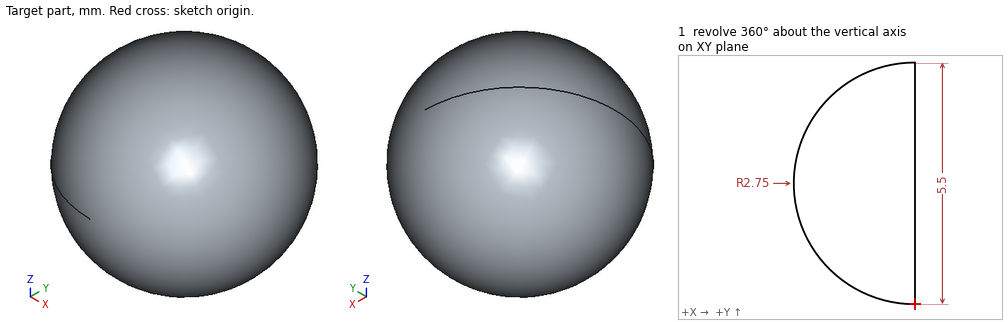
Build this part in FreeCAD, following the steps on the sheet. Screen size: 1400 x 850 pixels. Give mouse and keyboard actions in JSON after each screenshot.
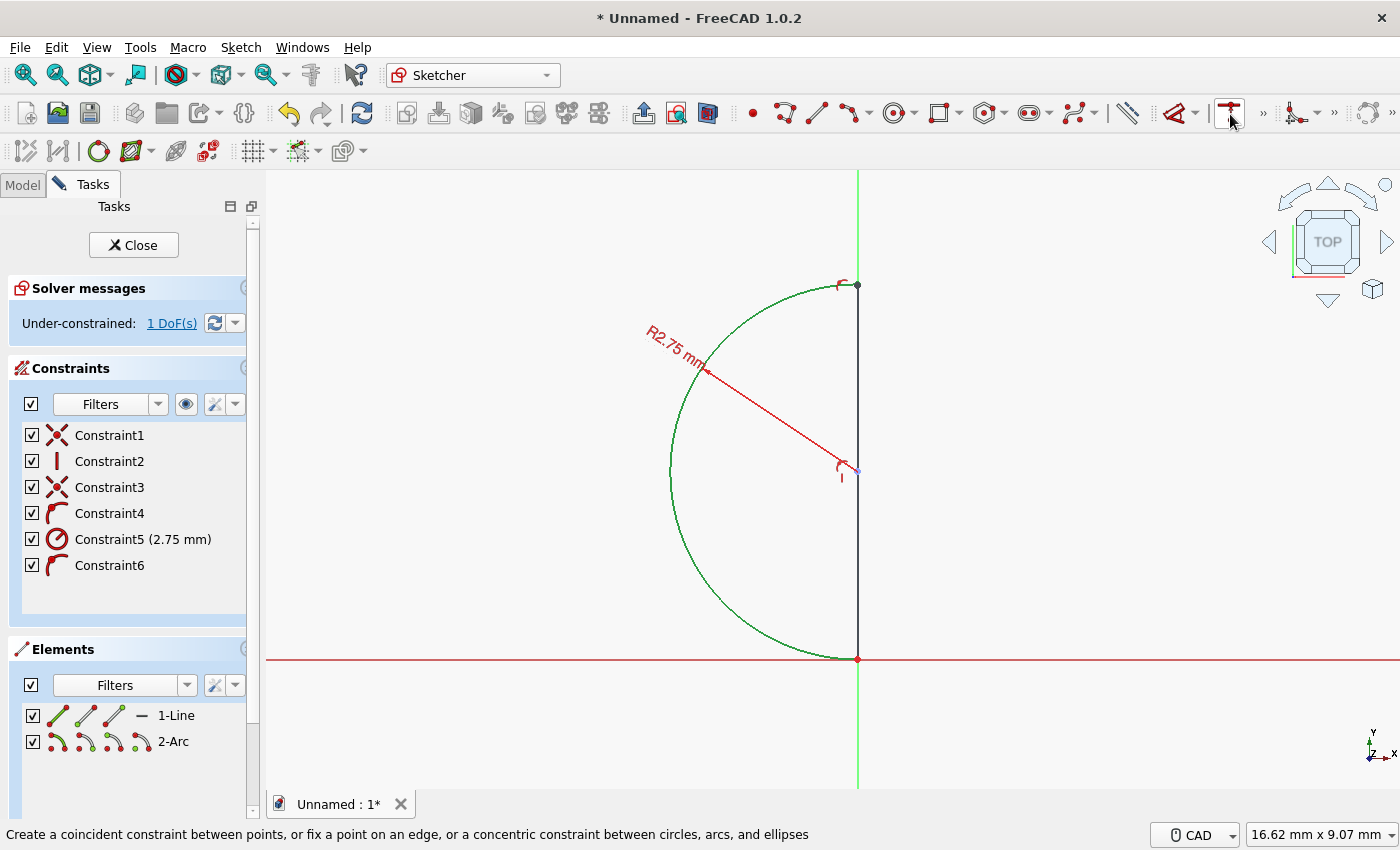
{"action": "left_click", "coordinate": [1174, 114]}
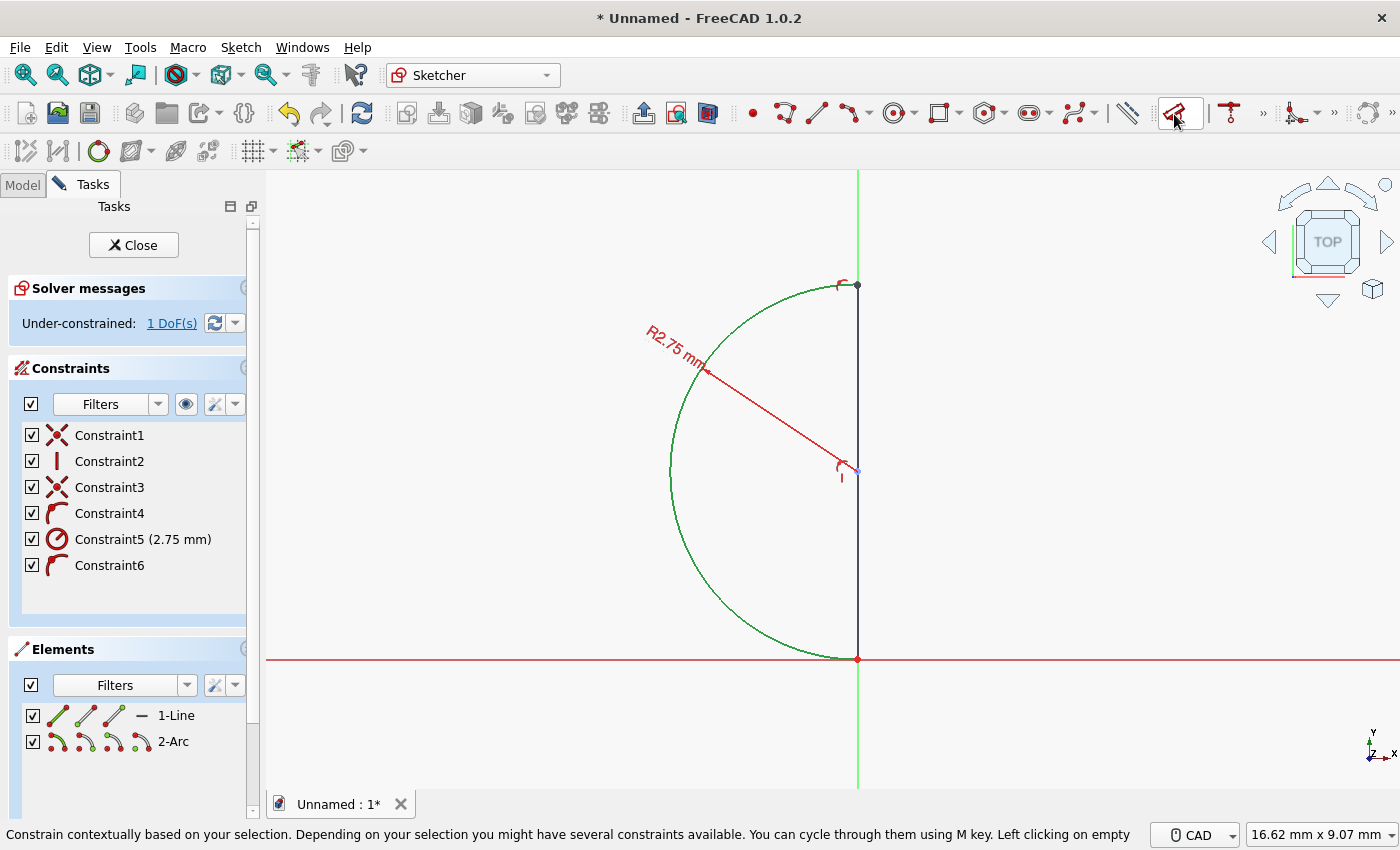
{"action": "left_click", "coordinate": [858, 547]}
{"action": "left_click", "coordinate": [892, 473]}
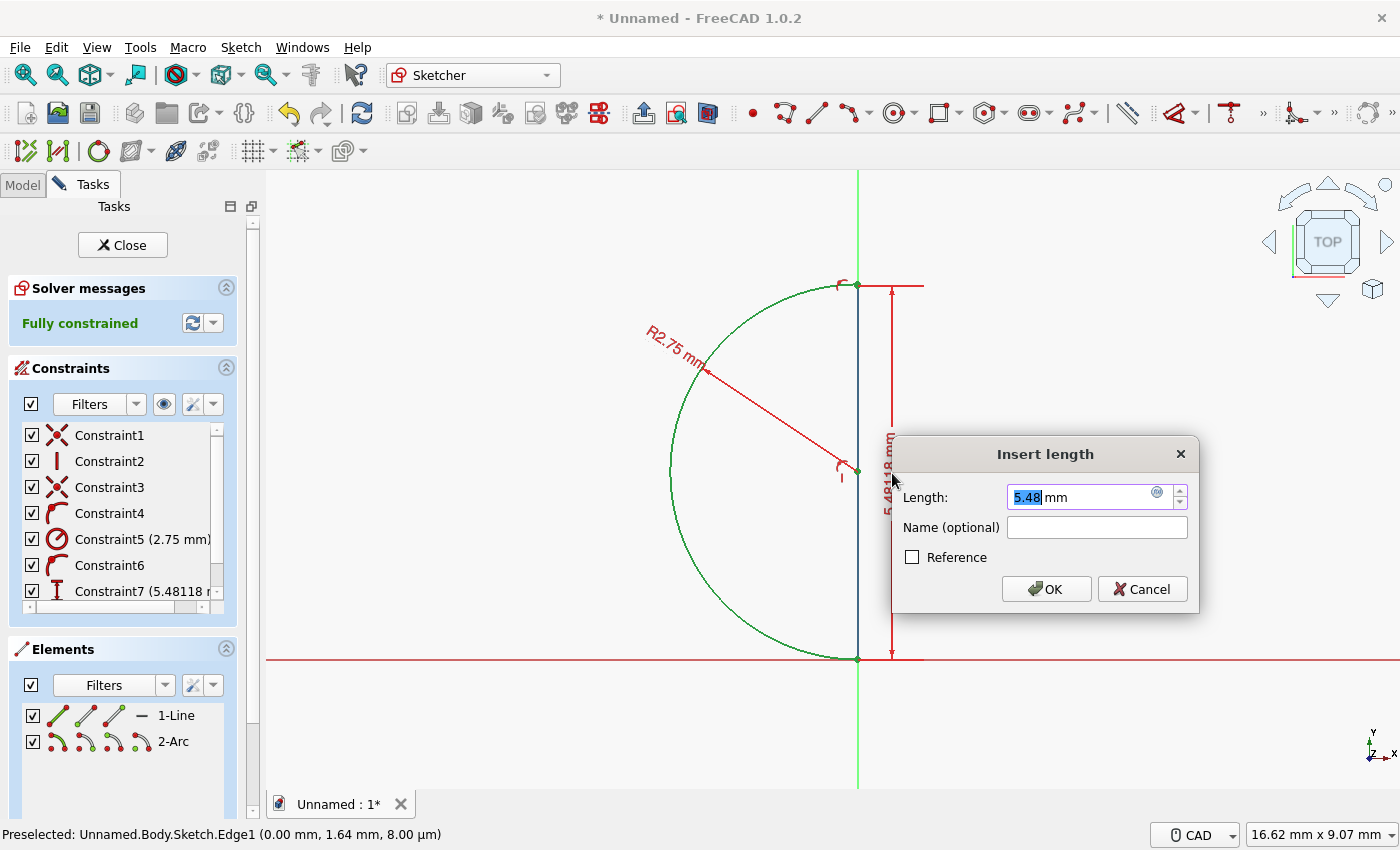
{"action": "type", "text": "5.5"}
{"action": "key", "text": "Return"}
{"action": "key", "text": "Escape"}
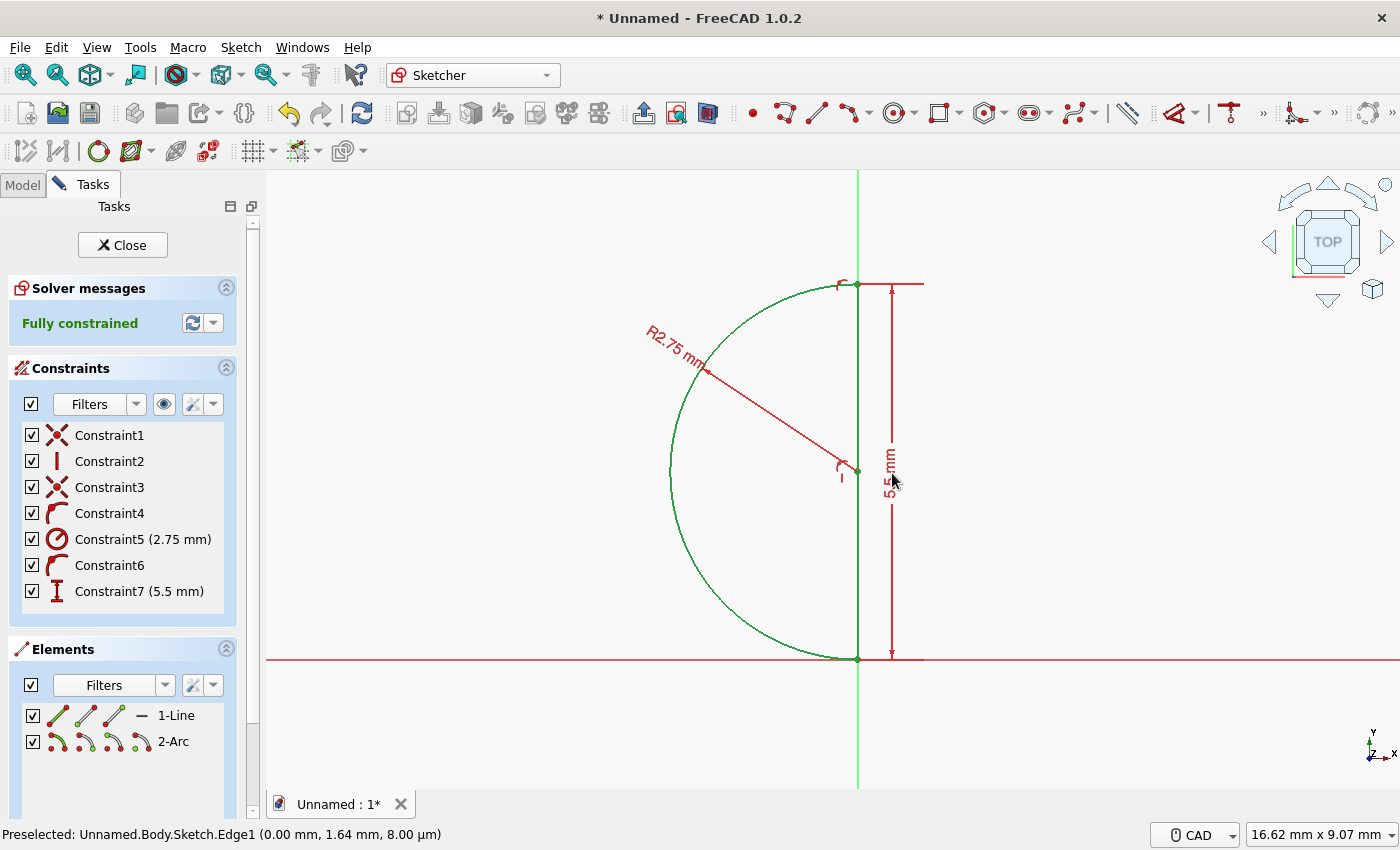
{"action": "left_click", "coordinate": [123, 245]}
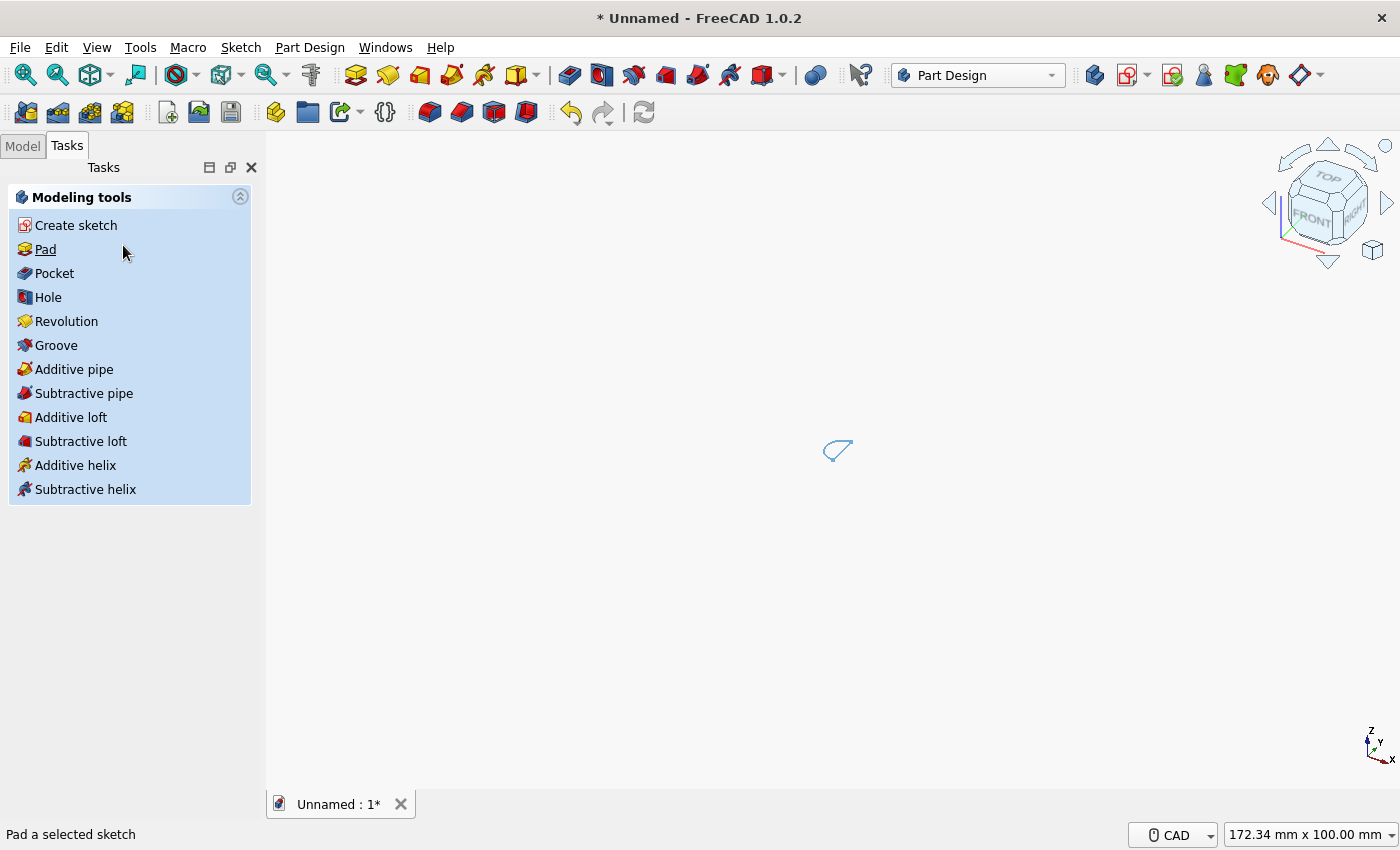
{"action": "left_click", "coordinate": [388, 76]}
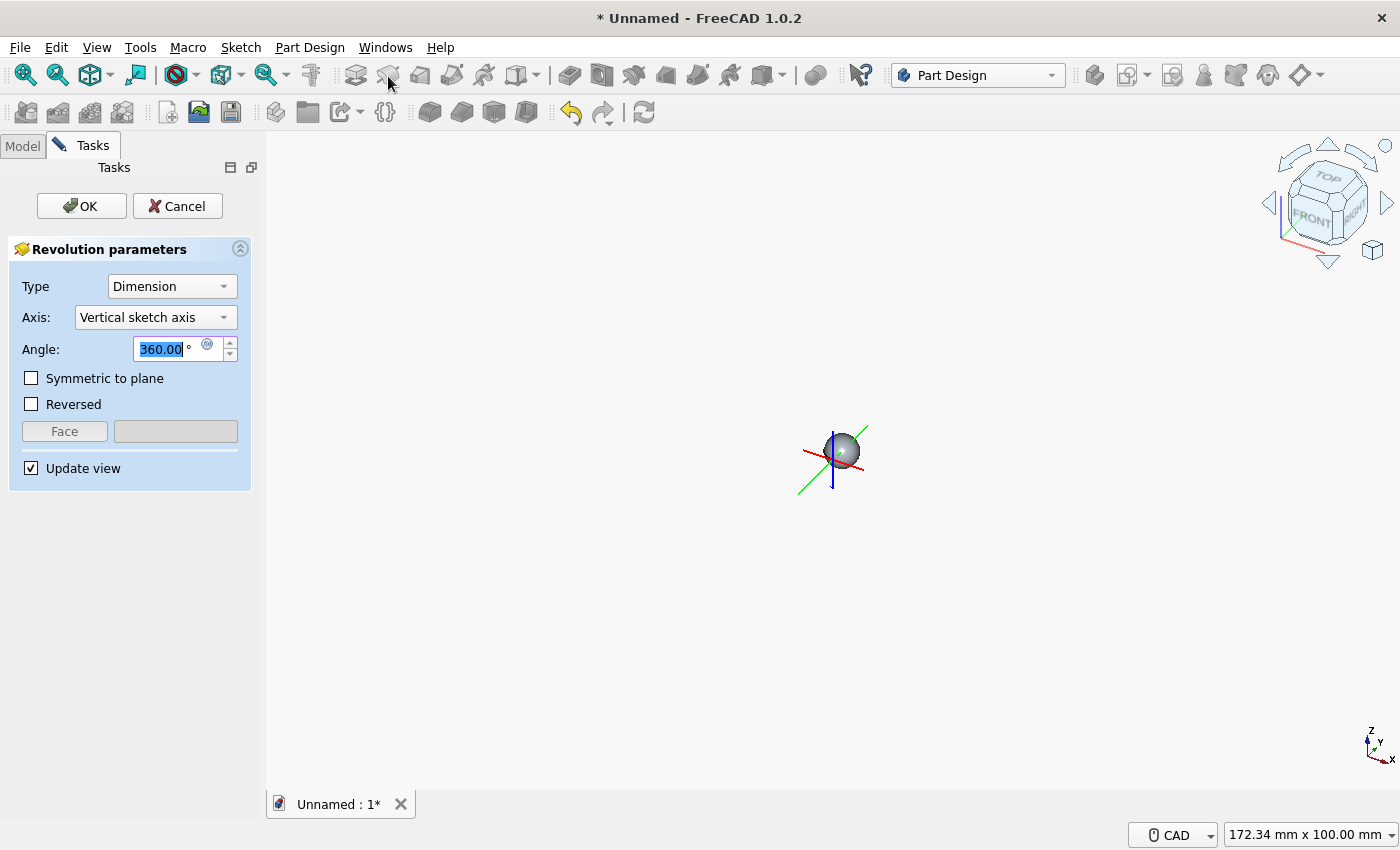
{"action": "left_click", "coordinate": [82, 206]}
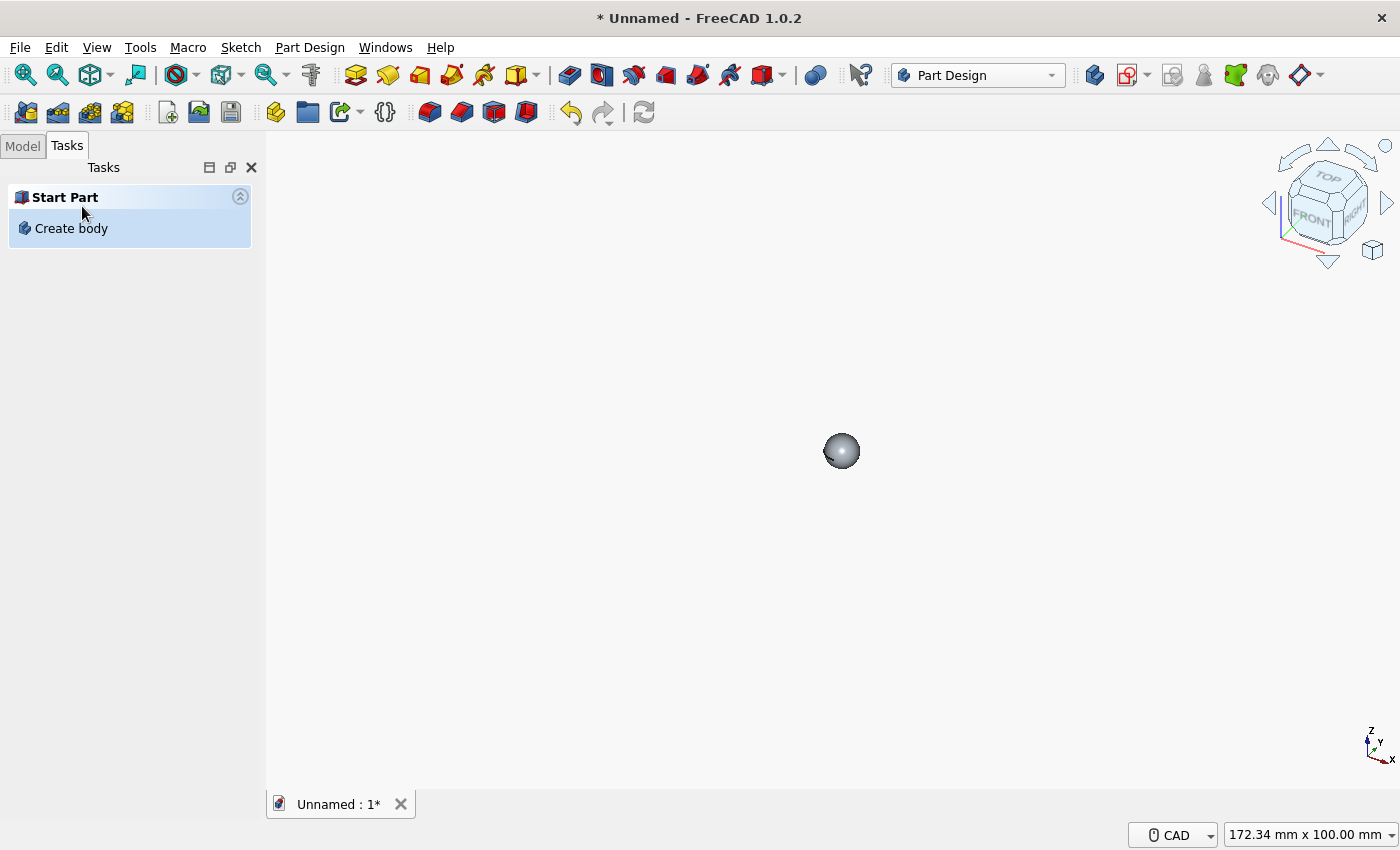
{"action": "key", "text": "0"}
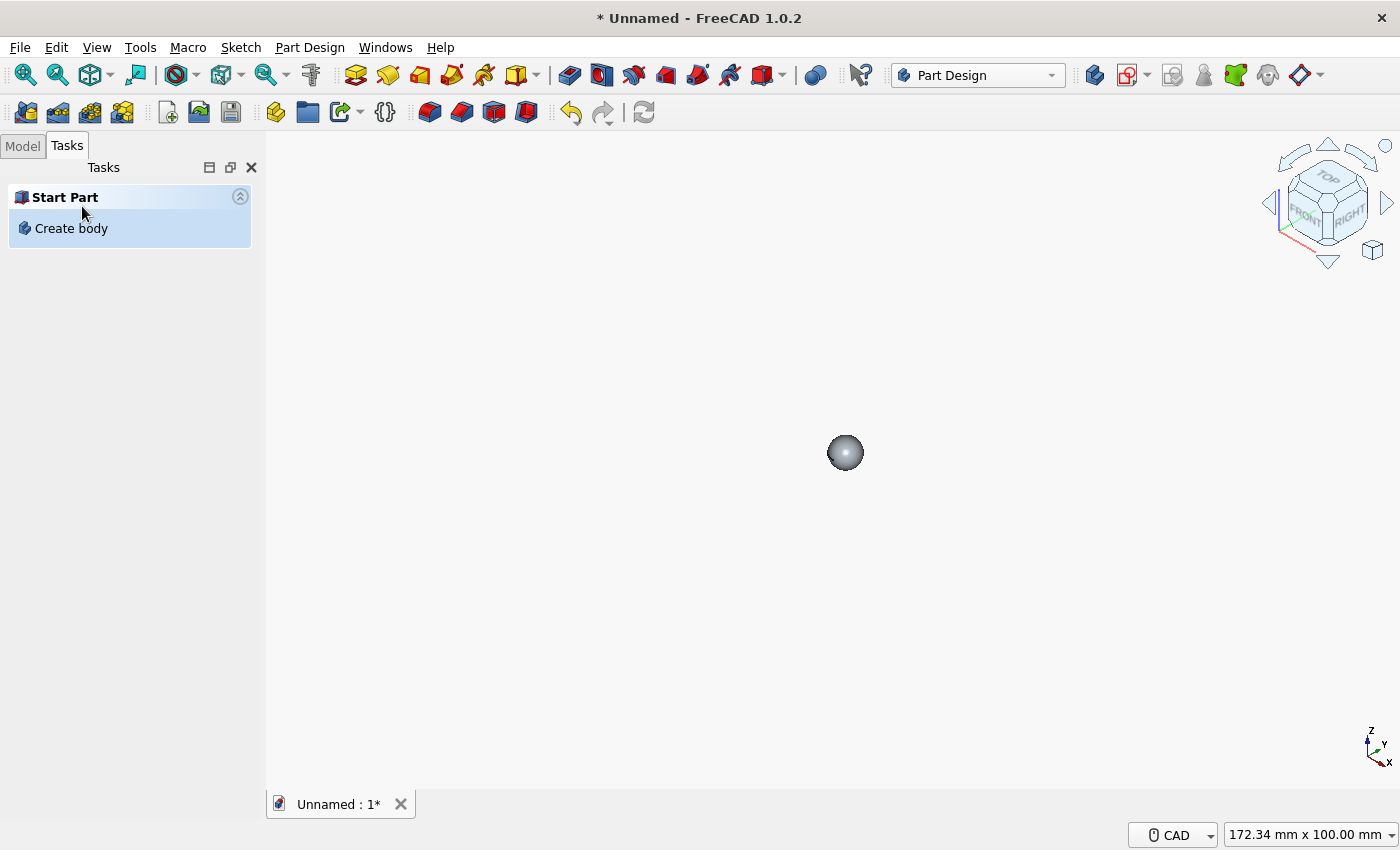
{"action": "left_click", "coordinate": [26, 76]}